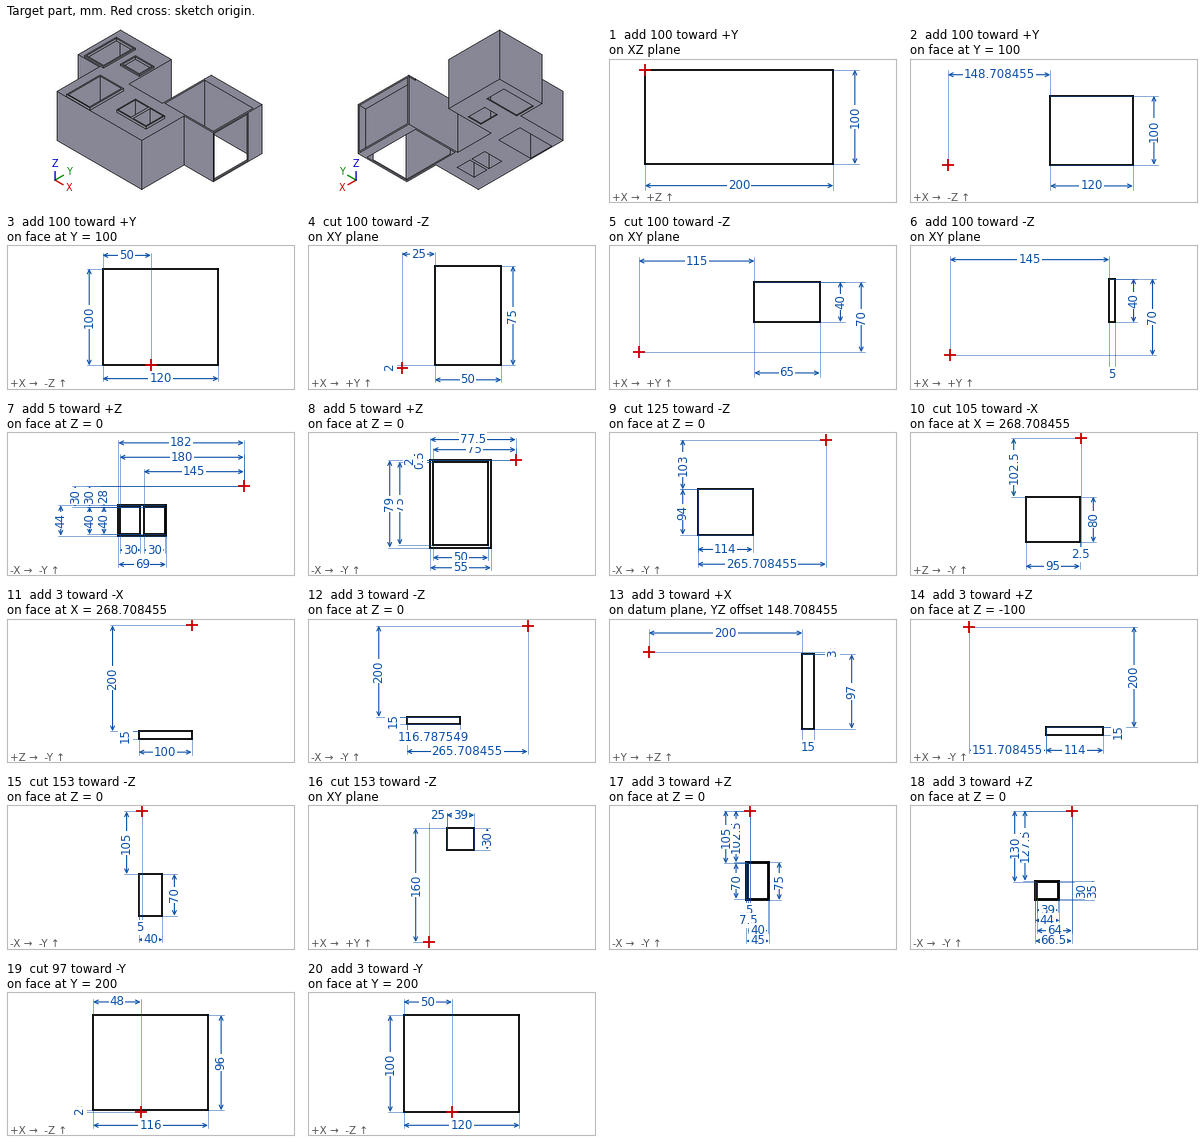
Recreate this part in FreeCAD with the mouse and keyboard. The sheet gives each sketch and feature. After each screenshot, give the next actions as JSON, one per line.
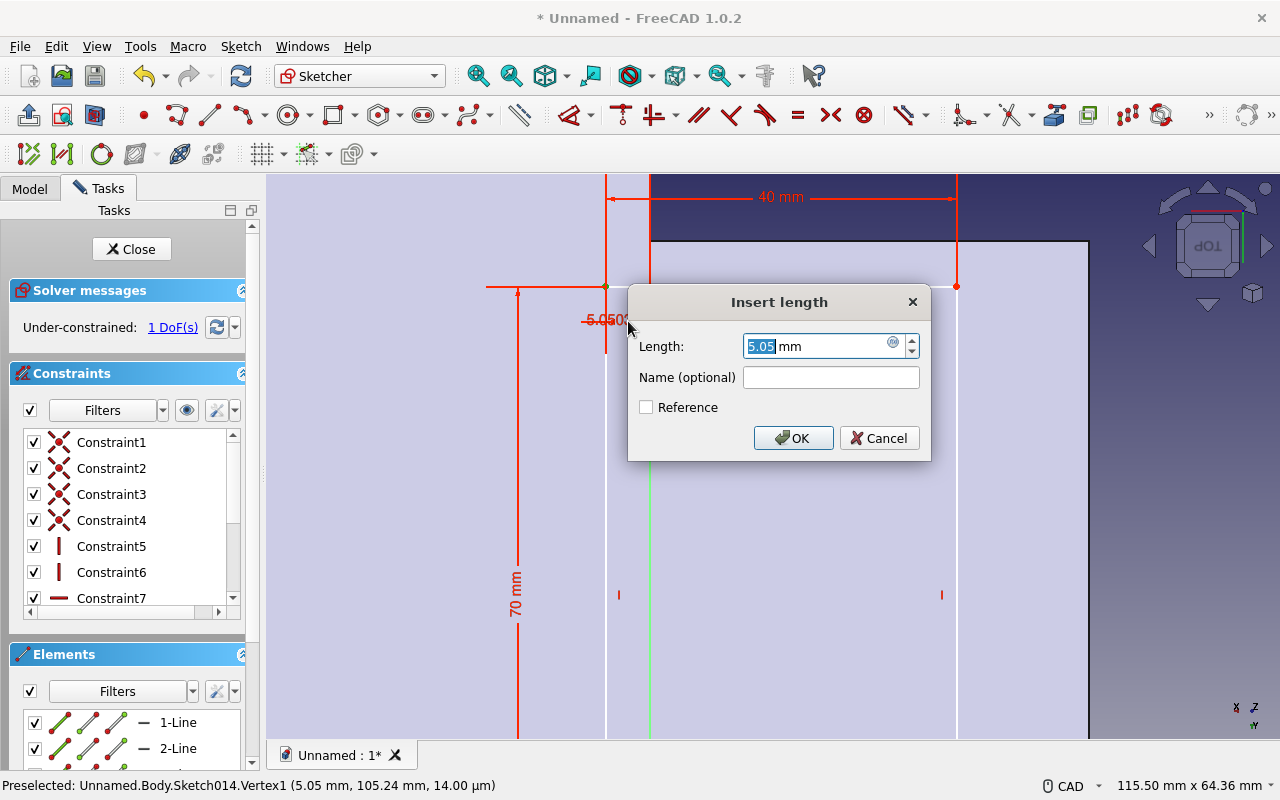
{"action": "type", "text": "5"}
{"action": "key", "text": "Return"}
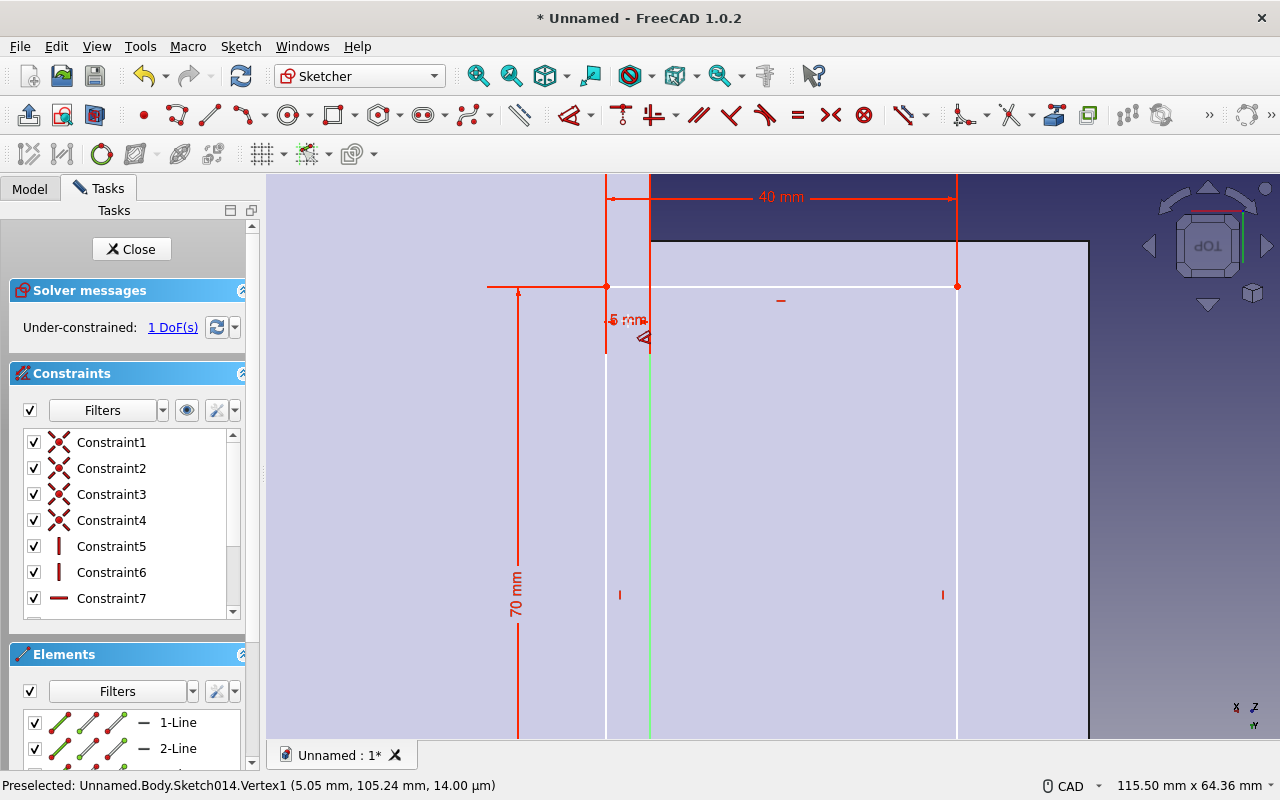
{"action": "left_click", "coordinate": [606, 287]}
{"action": "left_click", "coordinate": [572, 244]}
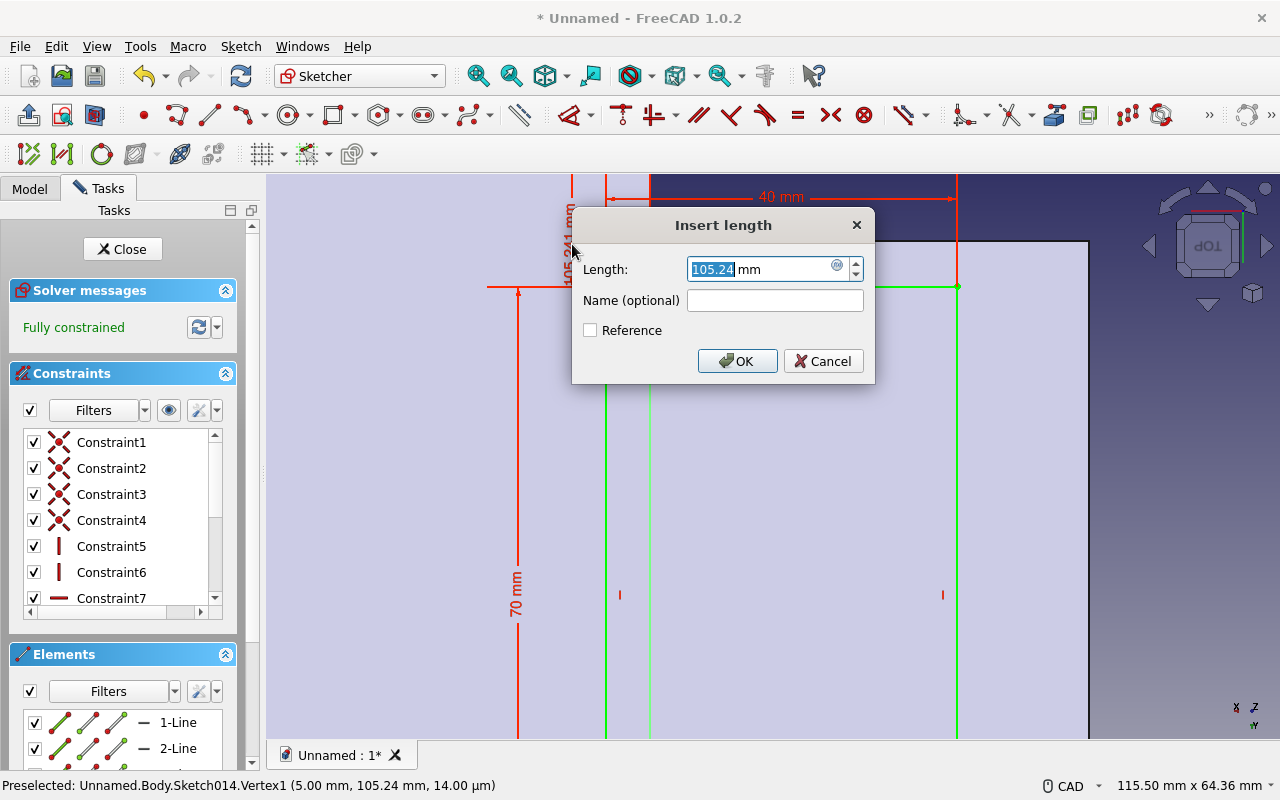
{"action": "type", "text": "105"}
{"action": "key", "text": "Return"}
{"action": "key", "text": "Escape"}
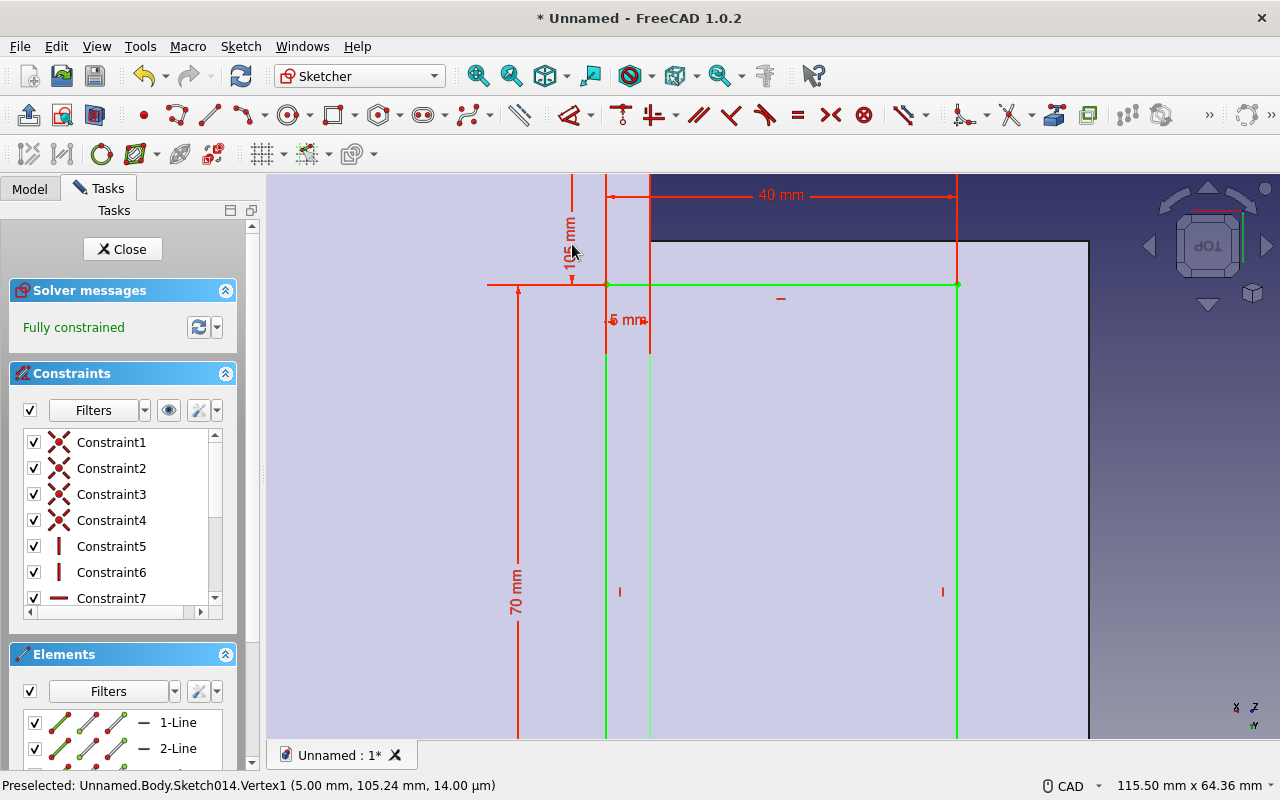
{"action": "left_click", "coordinate": [123, 249]}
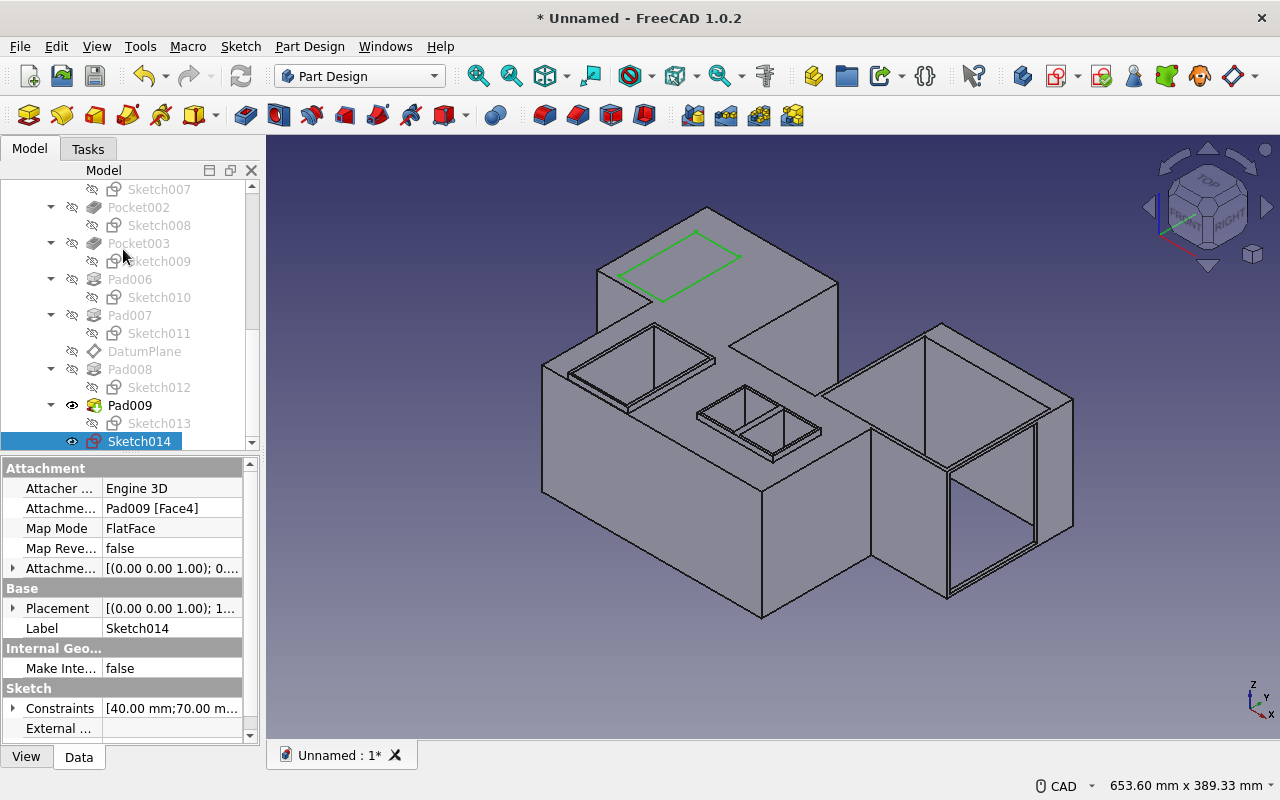
{"action": "left_click", "coordinate": [246, 116]}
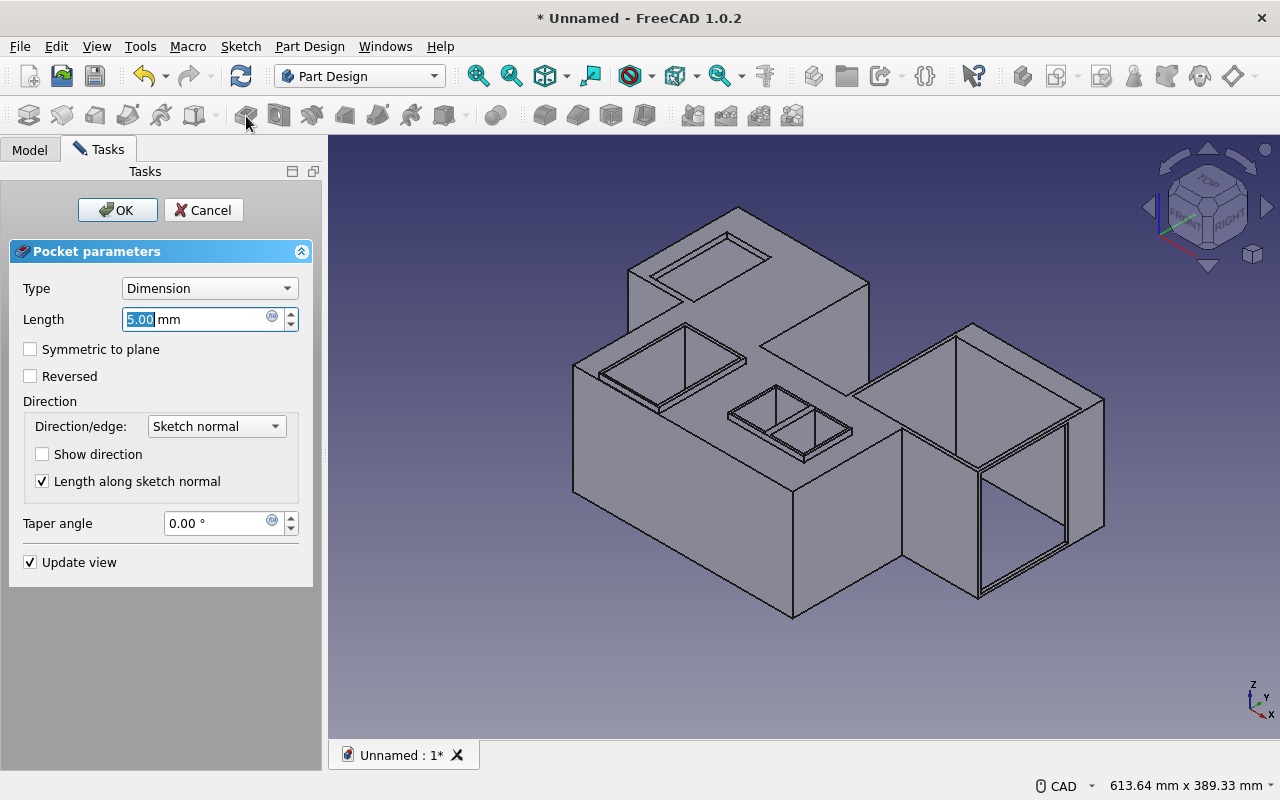
{"action": "type", "text": "153"}
{"action": "key", "text": "Tab"}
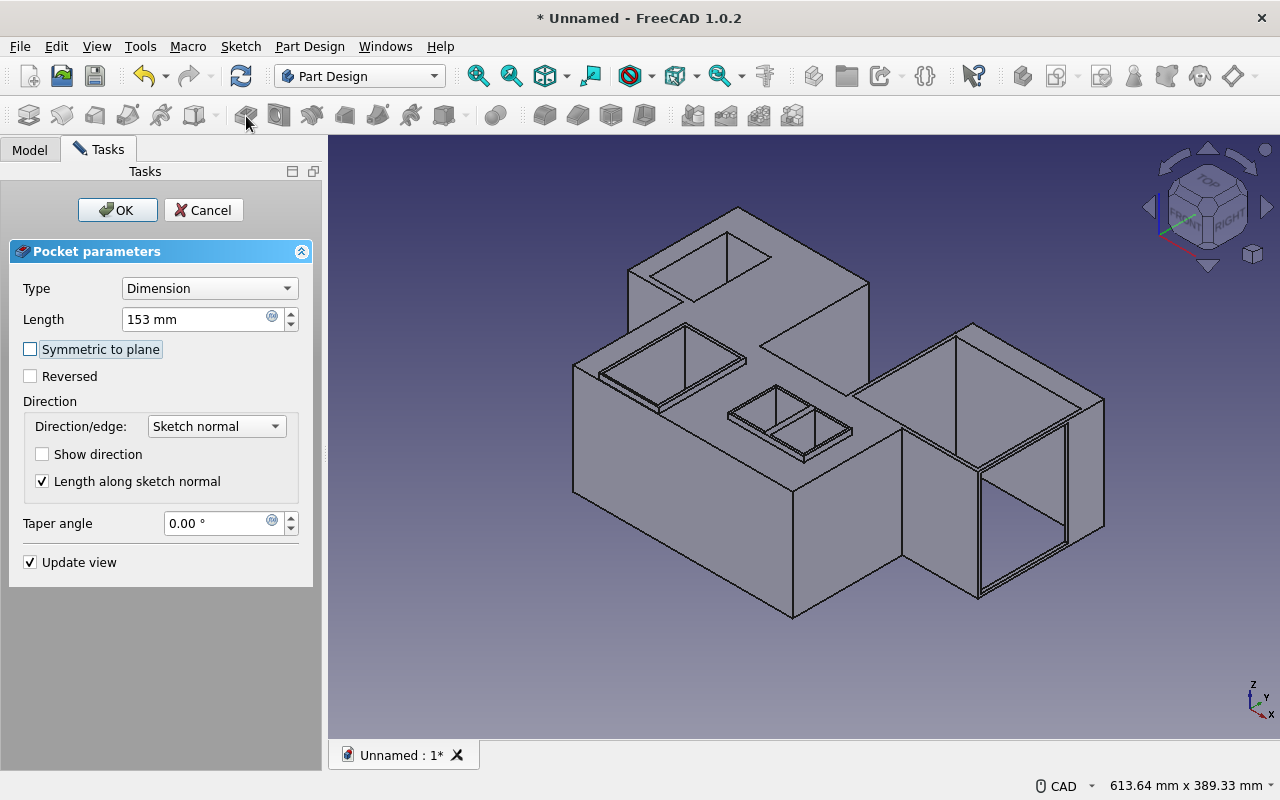
{"action": "left_click", "coordinate": [118, 210]}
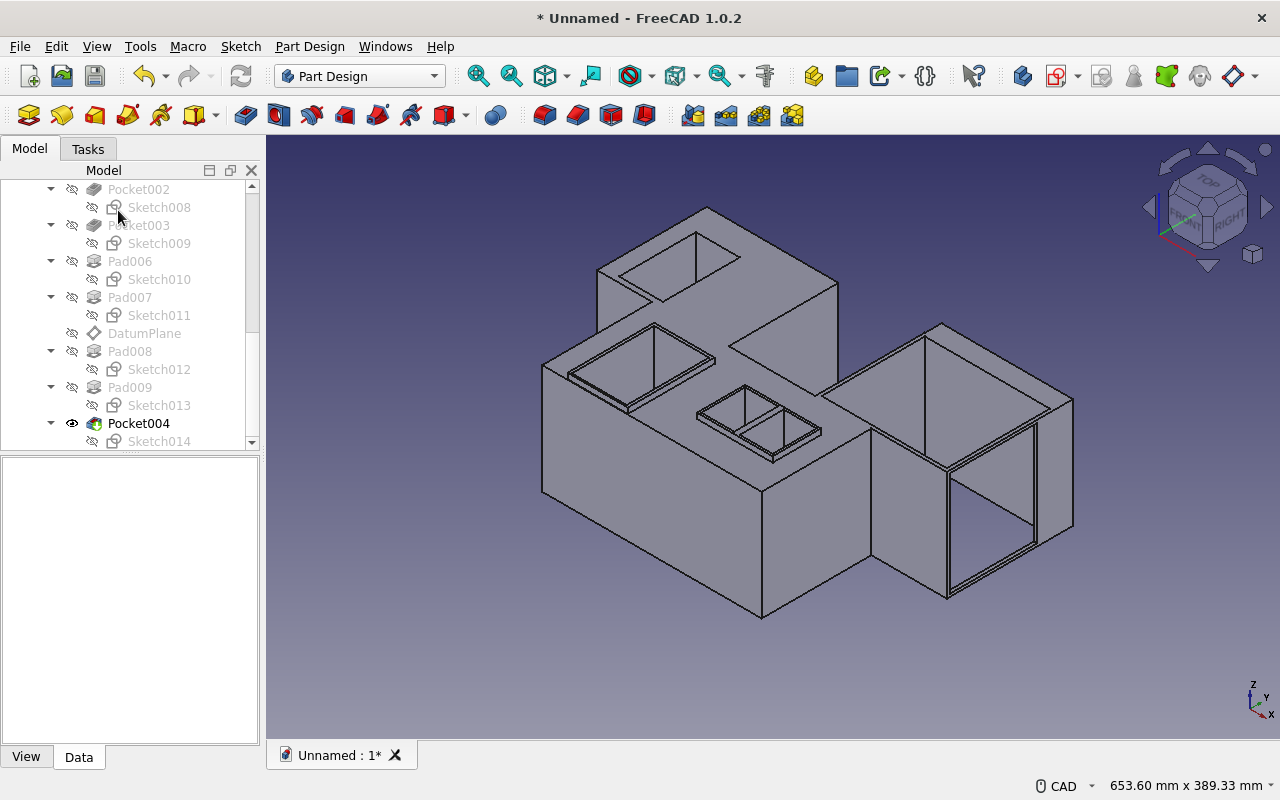
{"action": "left_click", "coordinate": [1056, 76]}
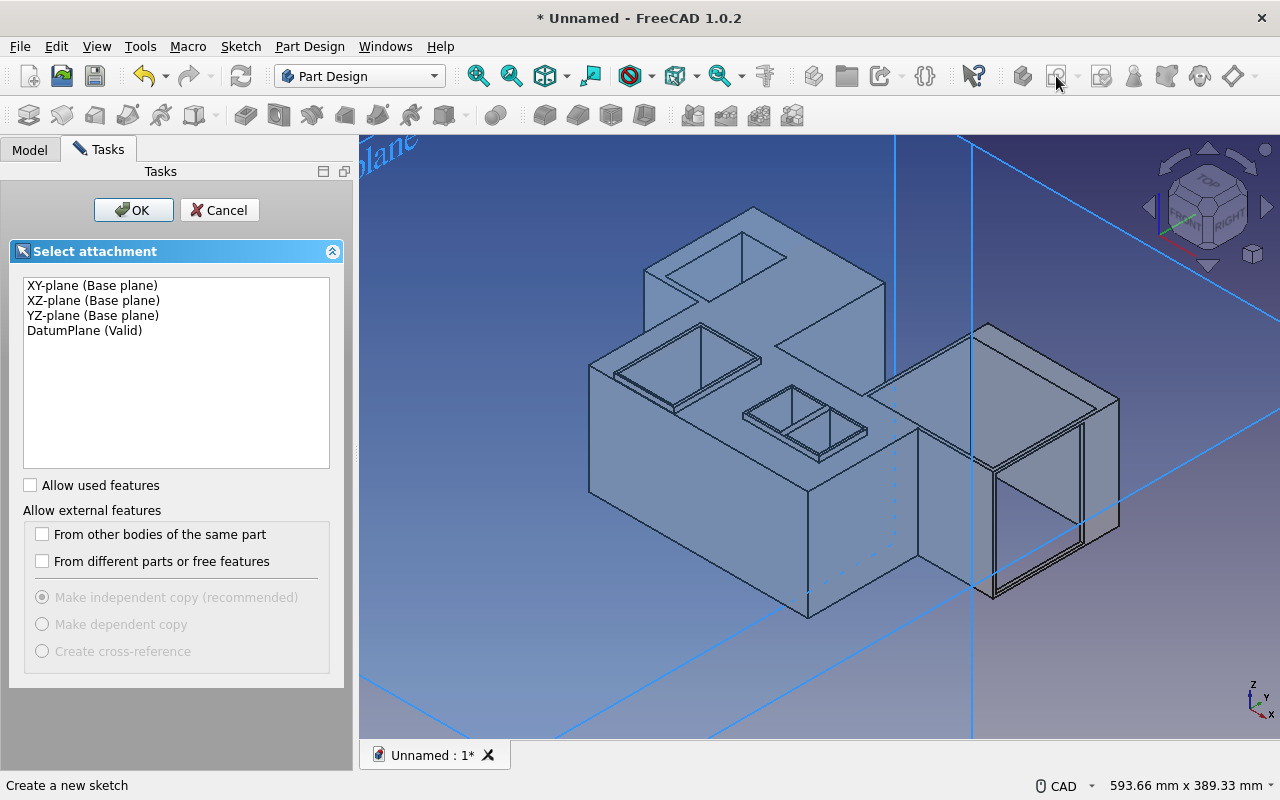
{"action": "left_click", "coordinate": [84, 286]}